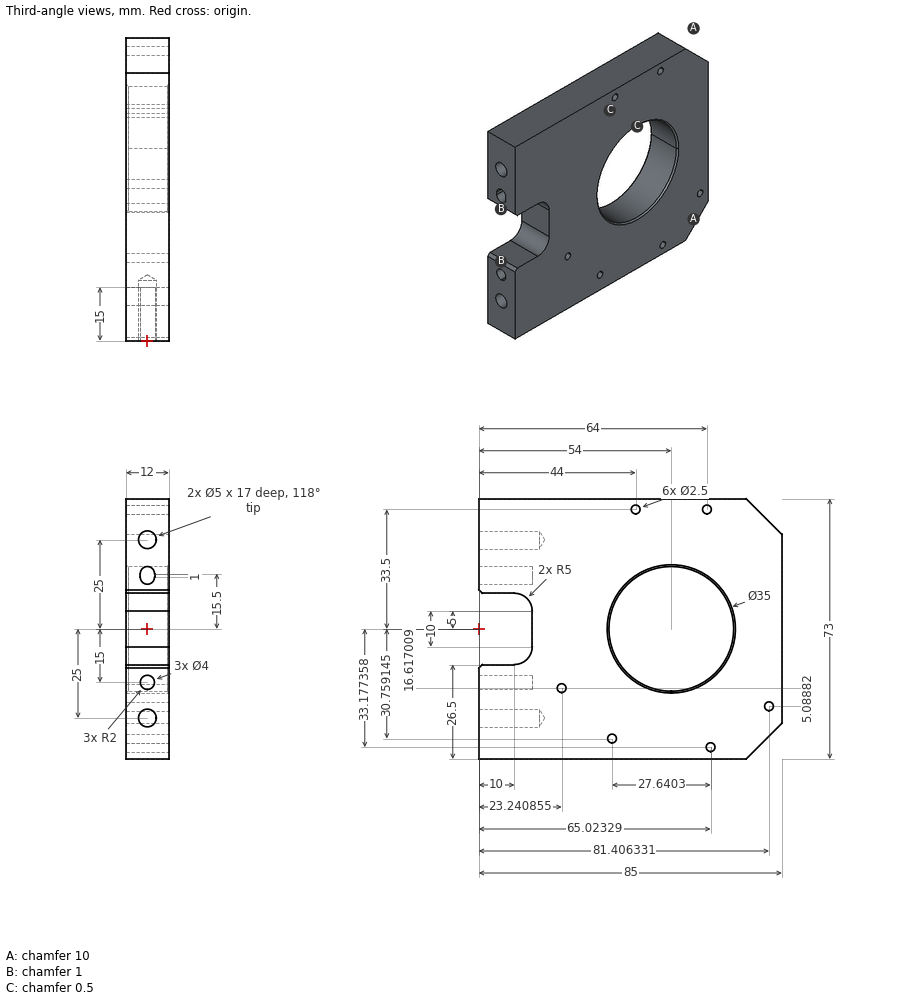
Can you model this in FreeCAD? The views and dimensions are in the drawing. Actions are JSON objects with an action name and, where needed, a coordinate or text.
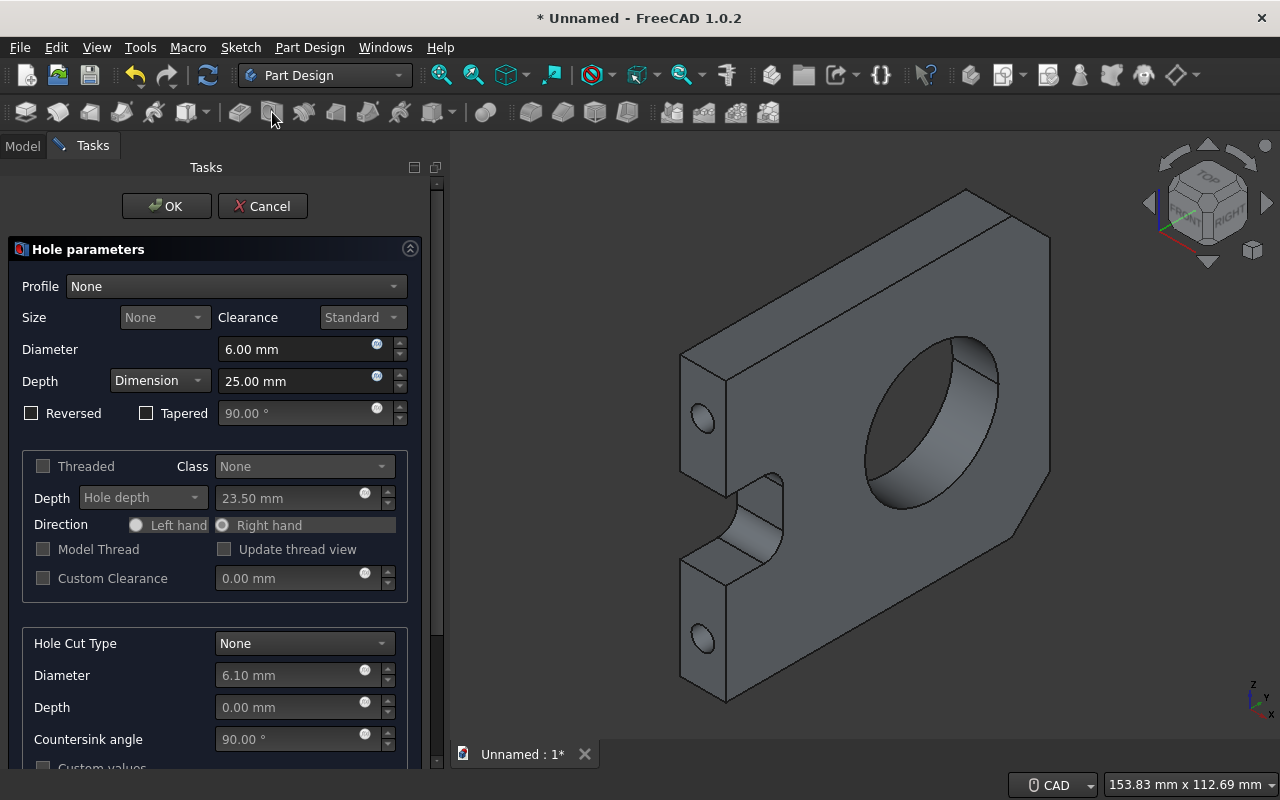
{"action": "triple_click", "coordinate": [305, 349]}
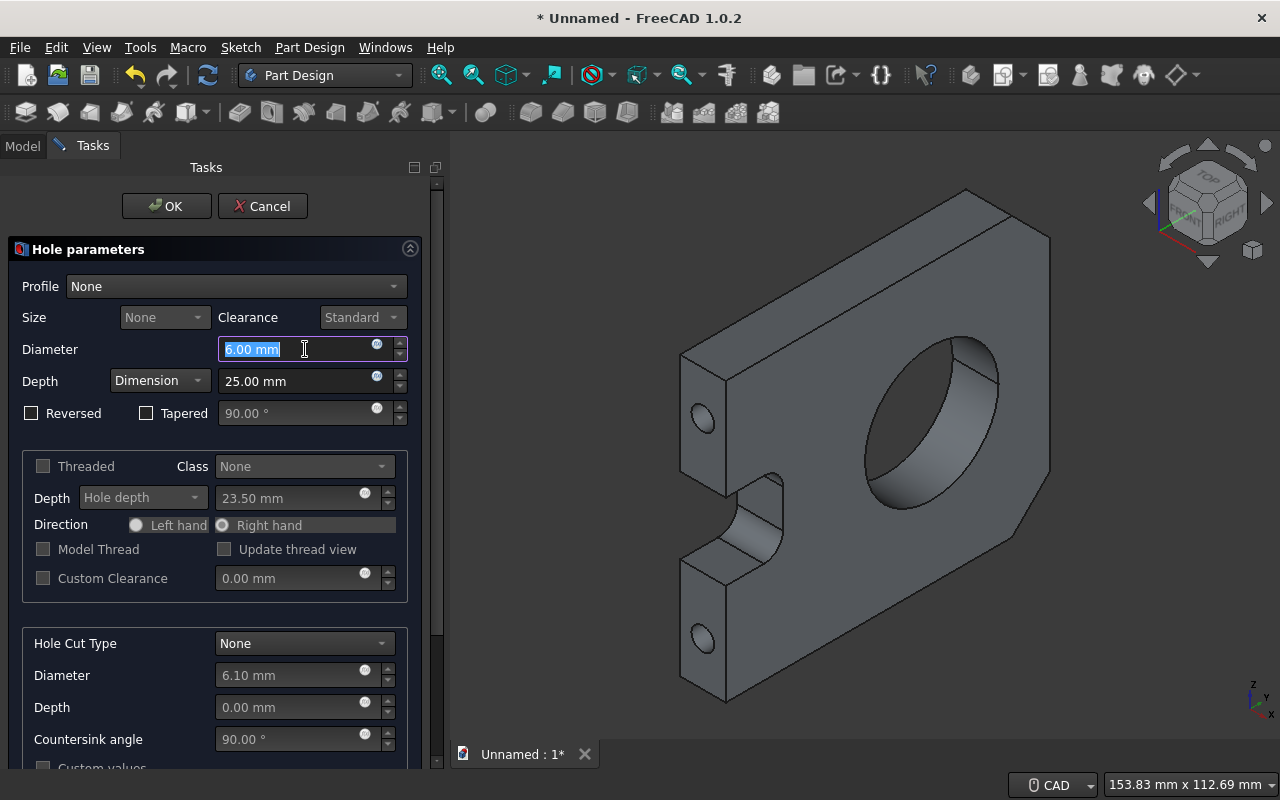
{"action": "type", "text": "5"}
{"action": "key", "text": "Tab"}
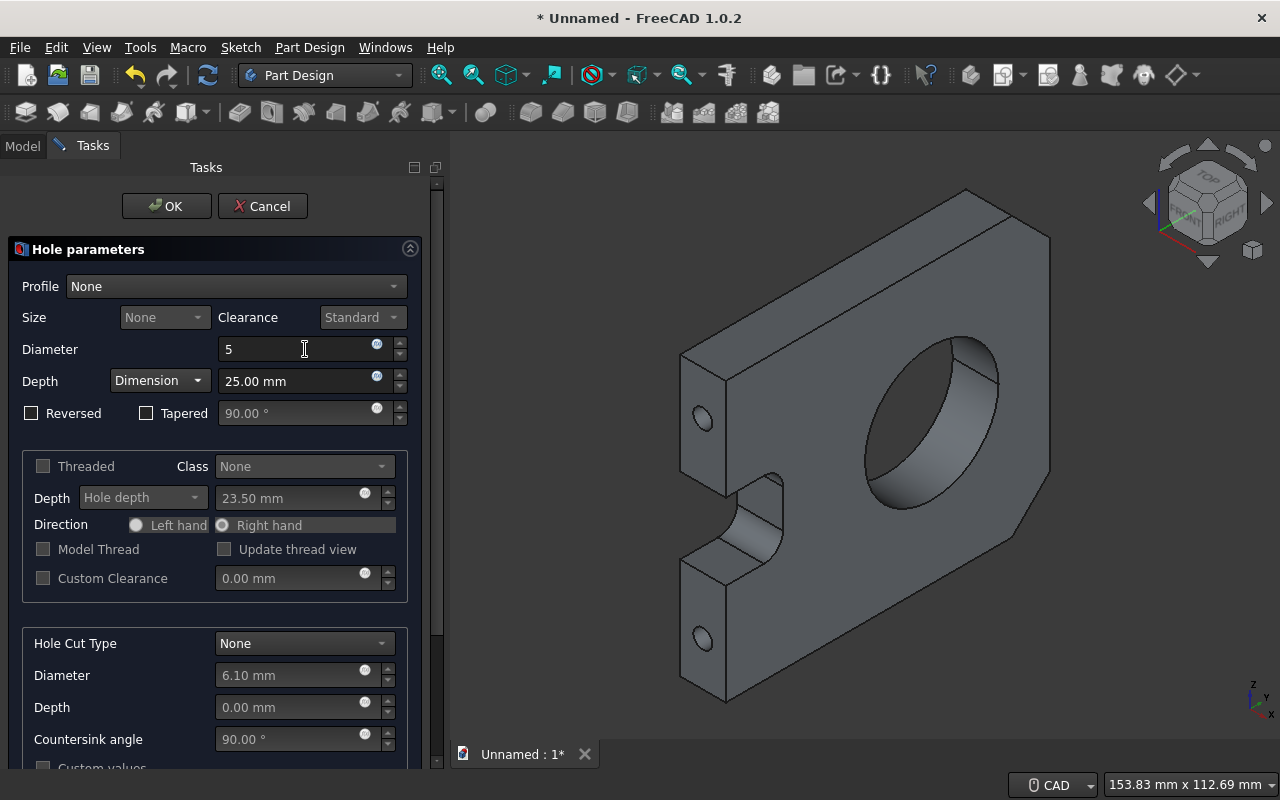
{"action": "triple_click", "coordinate": [305, 381]}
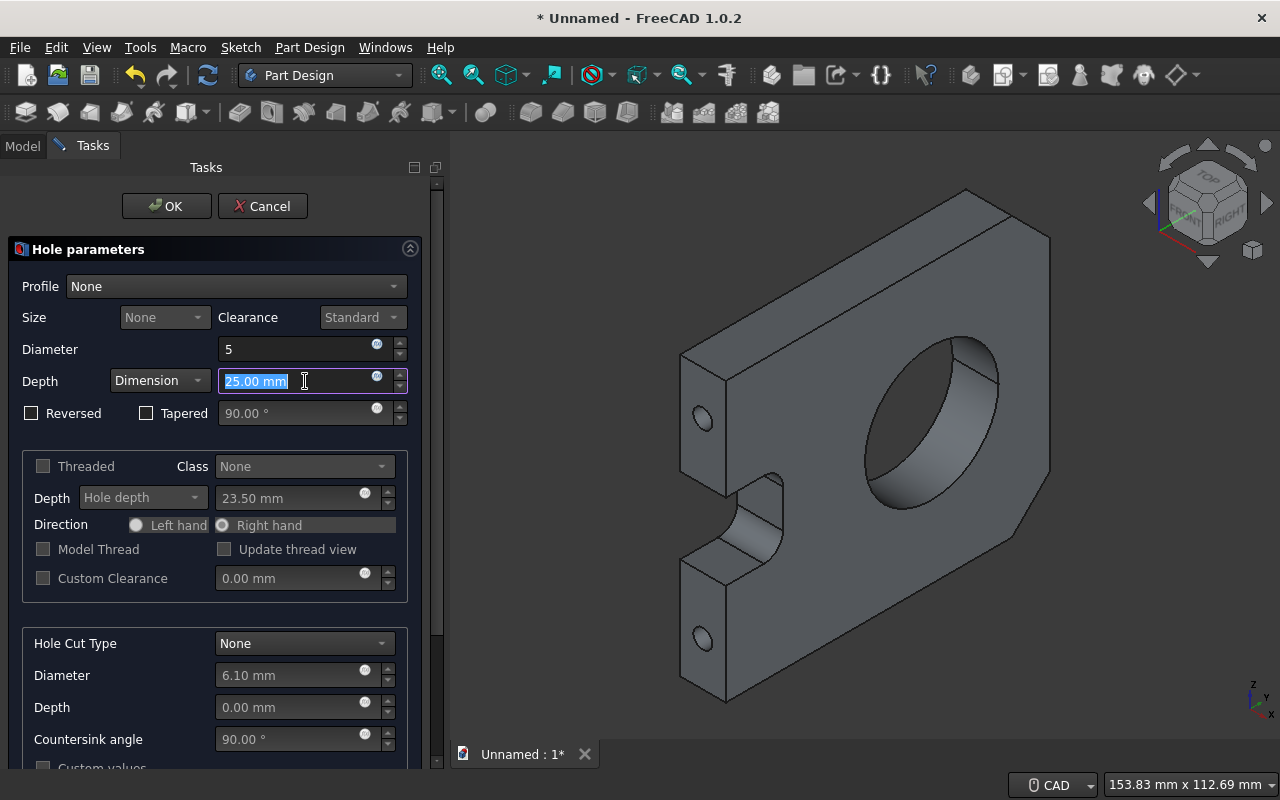
{"action": "type", "text": "17"}
{"action": "key", "text": "Tab"}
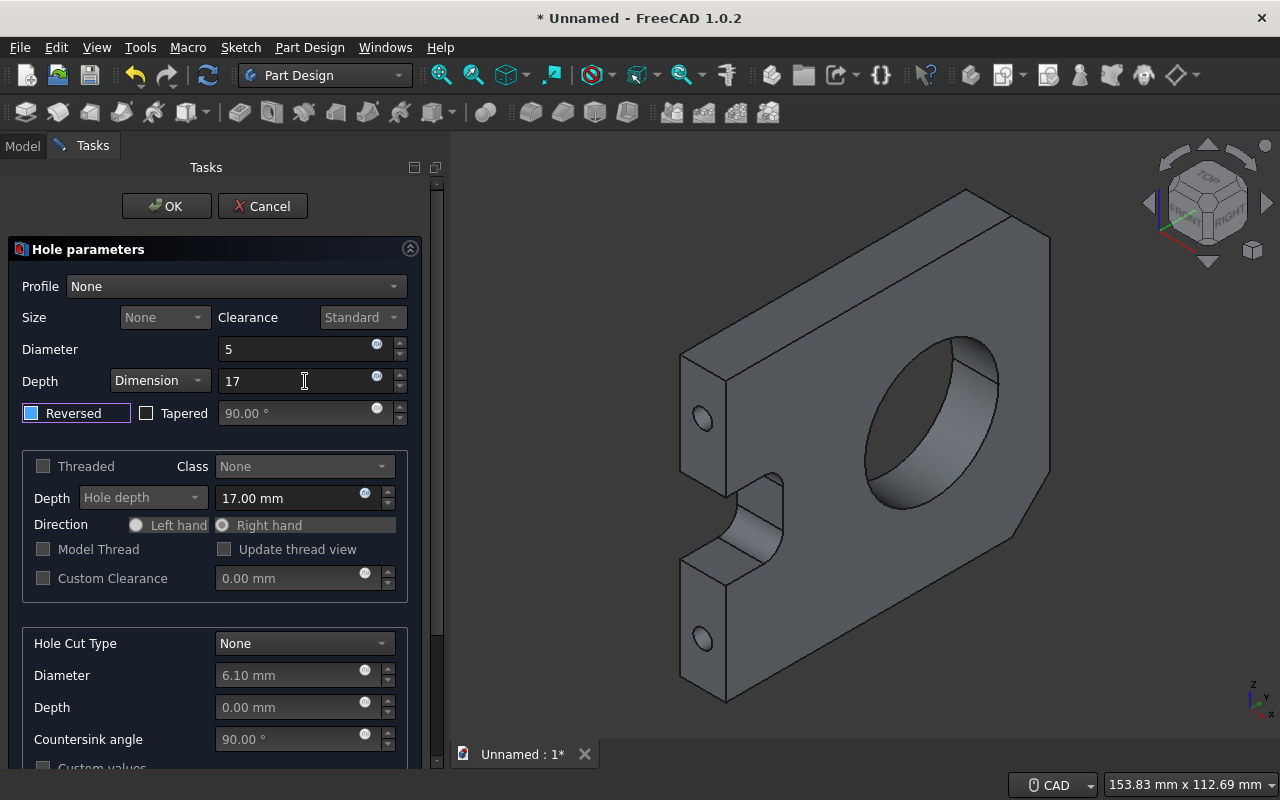
{"action": "left_click", "coordinate": [167, 206]}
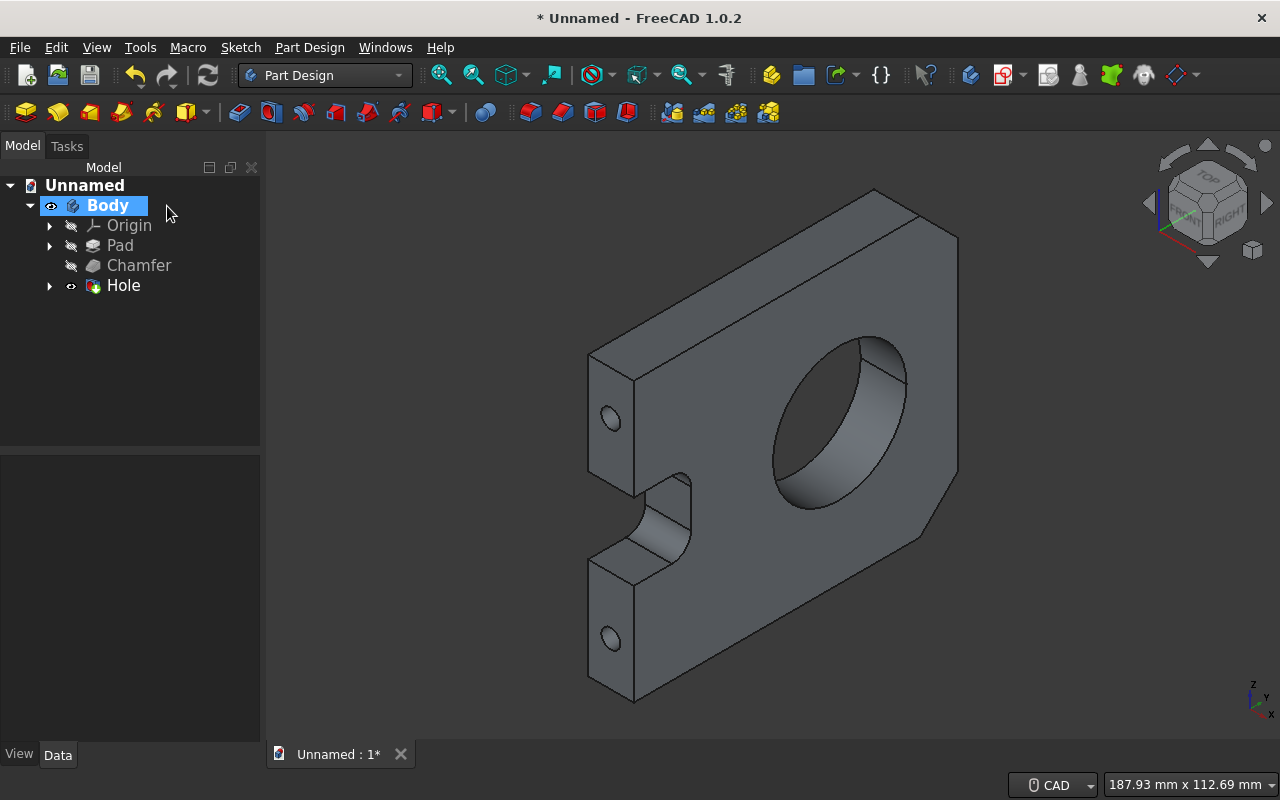
{"action": "left_click", "coordinate": [611, 597]}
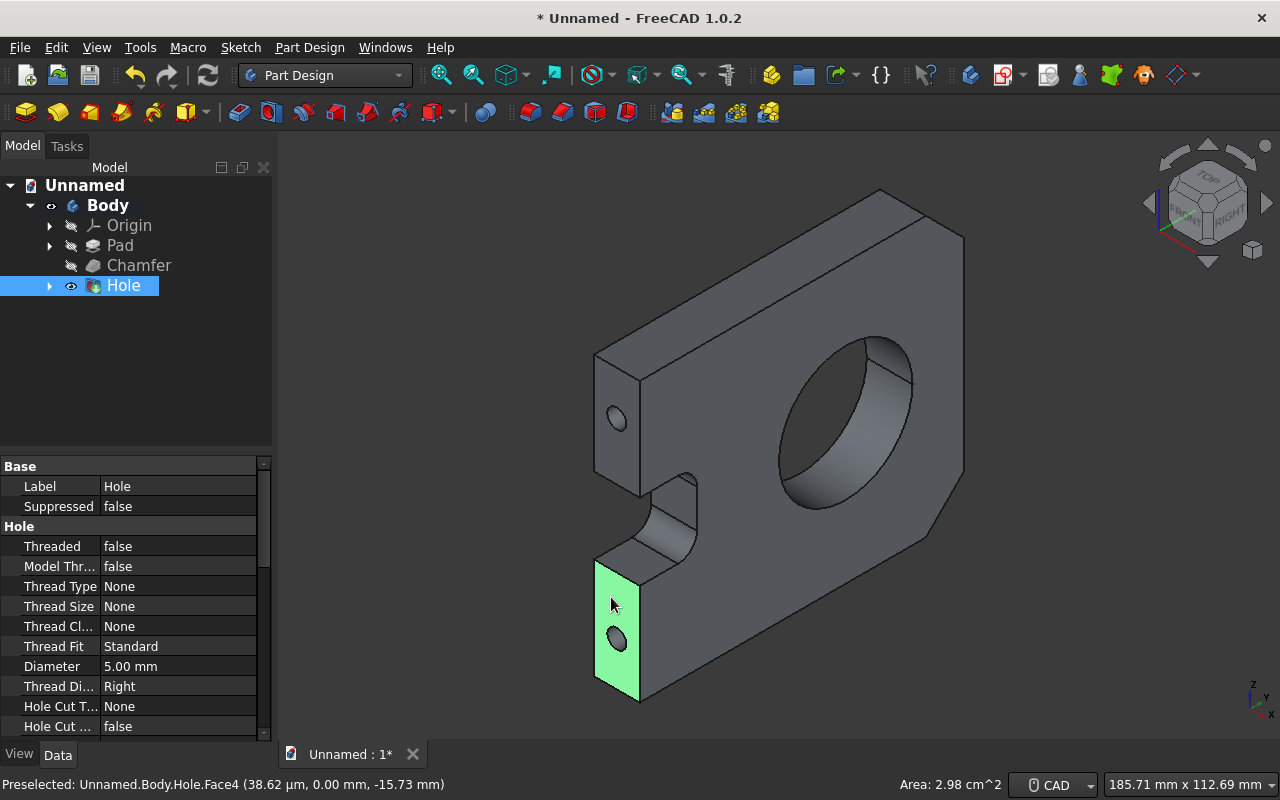
{"action": "left_click", "coordinate": [1004, 76]}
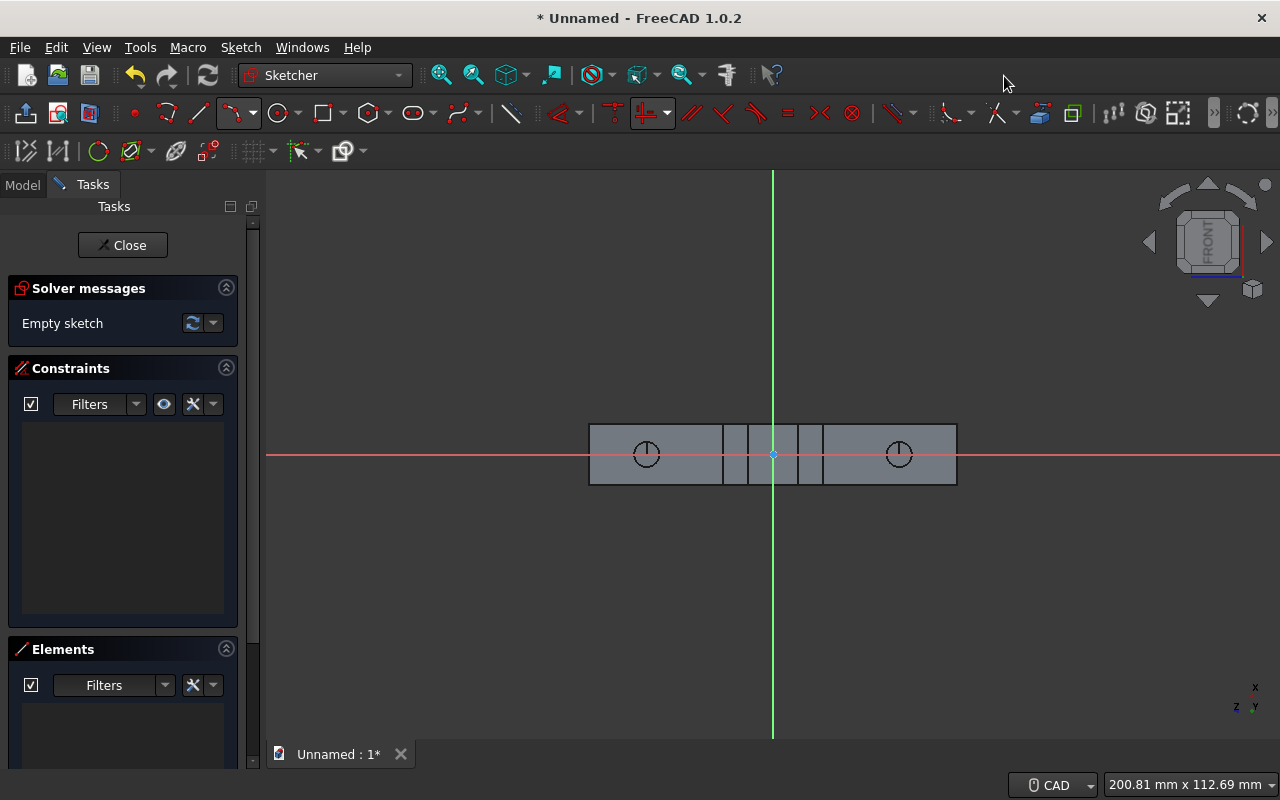
{"action": "scroll", "coordinate": [801, 455], "scroll_direction": "up", "scroll_amount": 6}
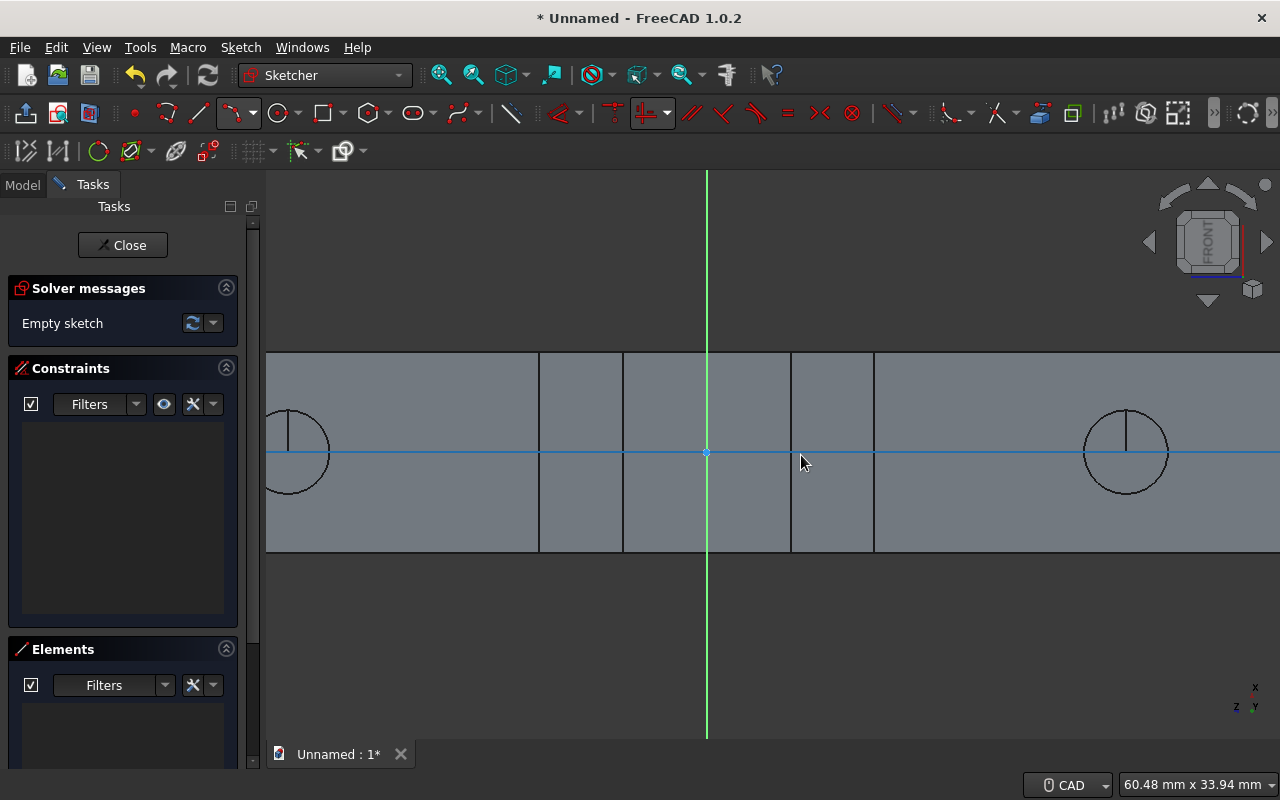
{"action": "left_click", "coordinate": [414, 114]}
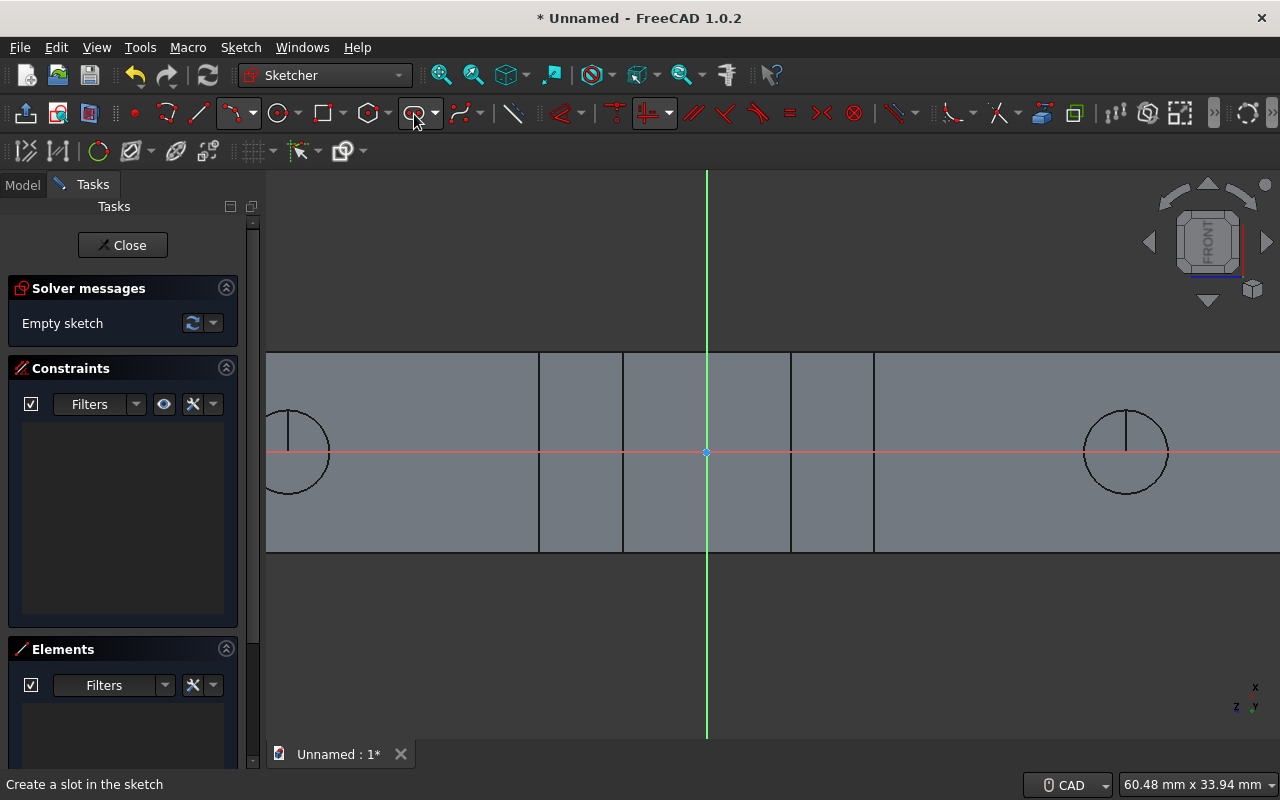
{"action": "left_click", "coordinate": [447, 452]}